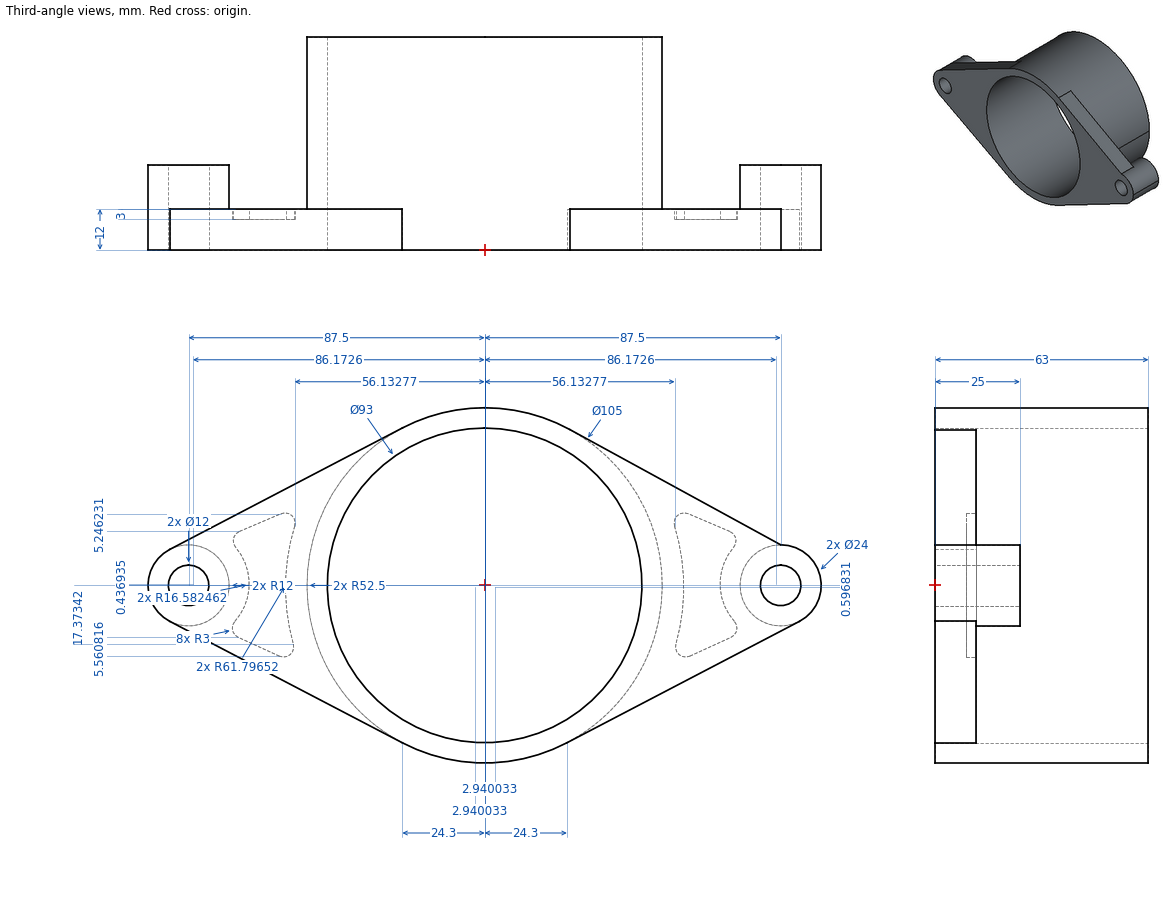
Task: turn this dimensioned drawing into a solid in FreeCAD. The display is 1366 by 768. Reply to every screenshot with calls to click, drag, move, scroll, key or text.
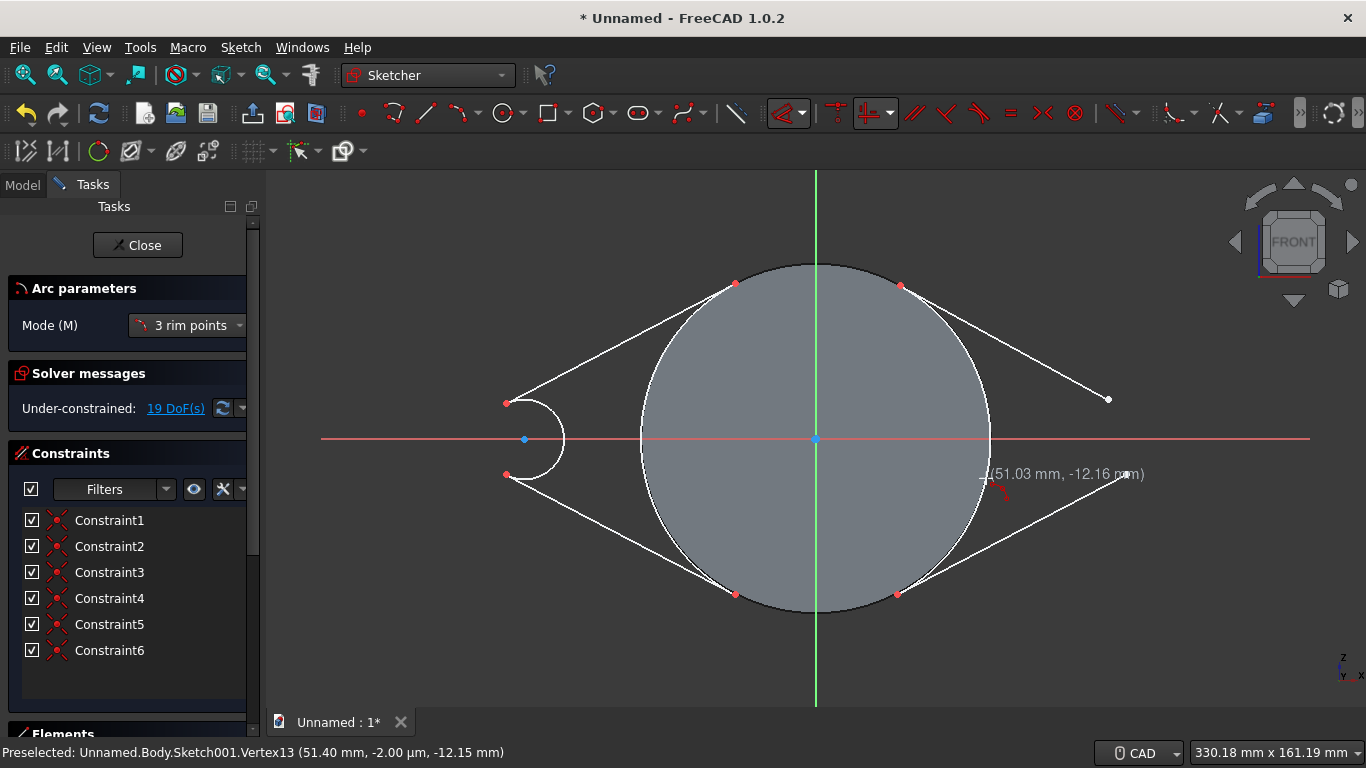
click(1108, 400)
click(1126, 475)
click(1075, 461)
key(Escape)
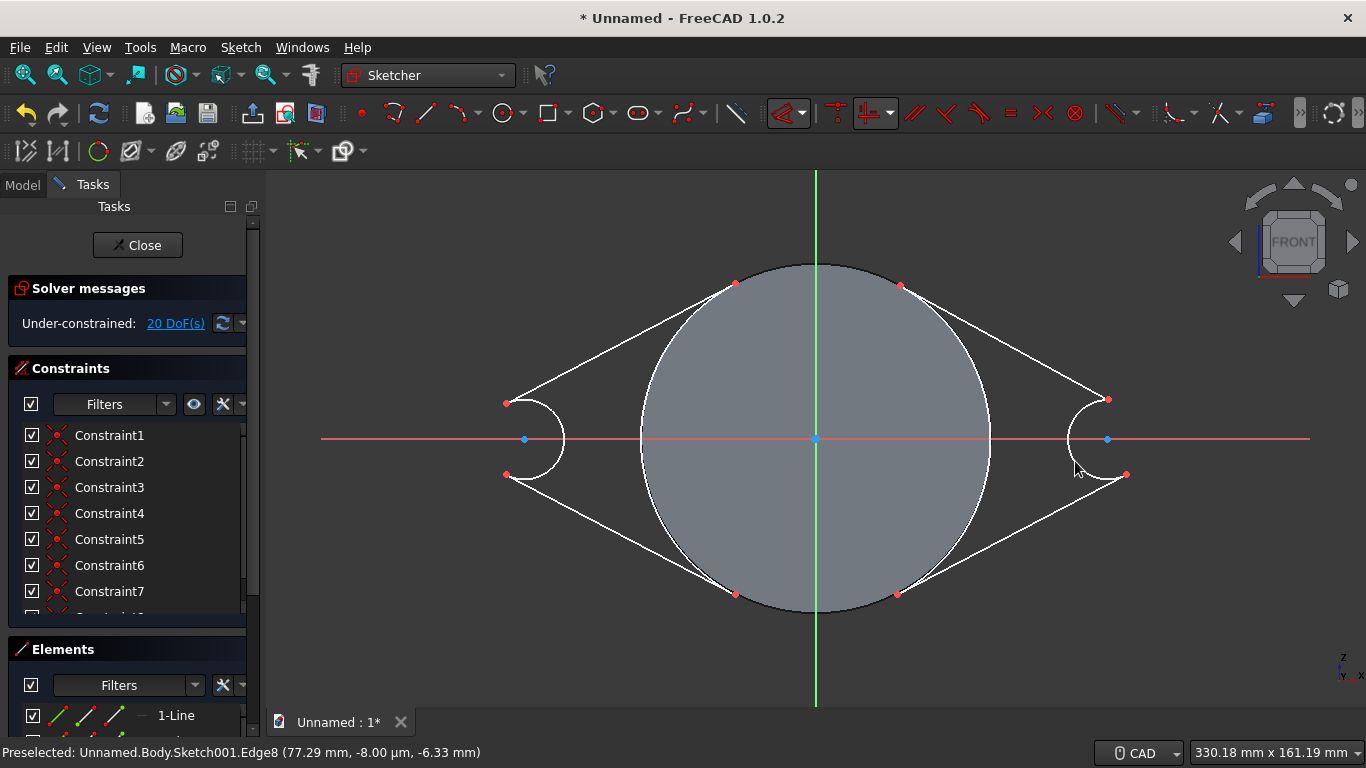
click(666, 559)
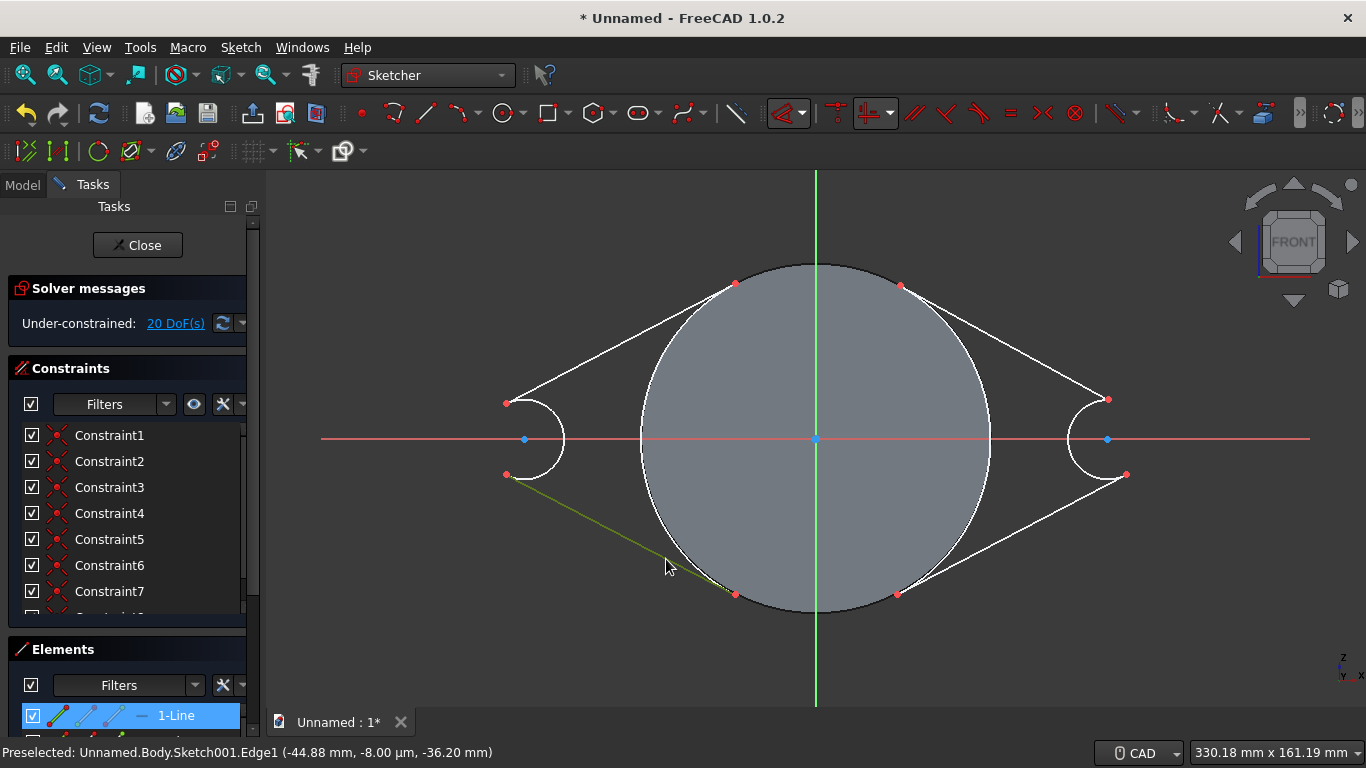
click(552, 469)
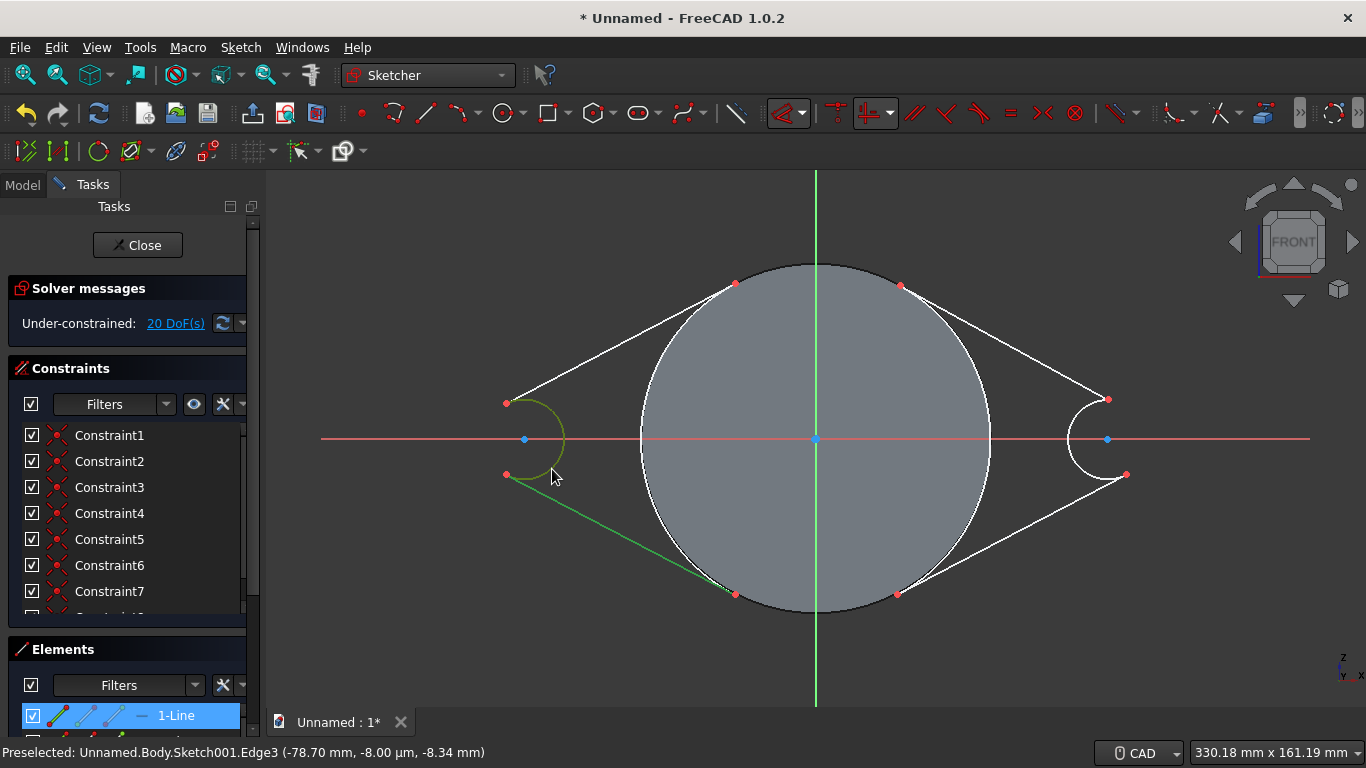
click(980, 114)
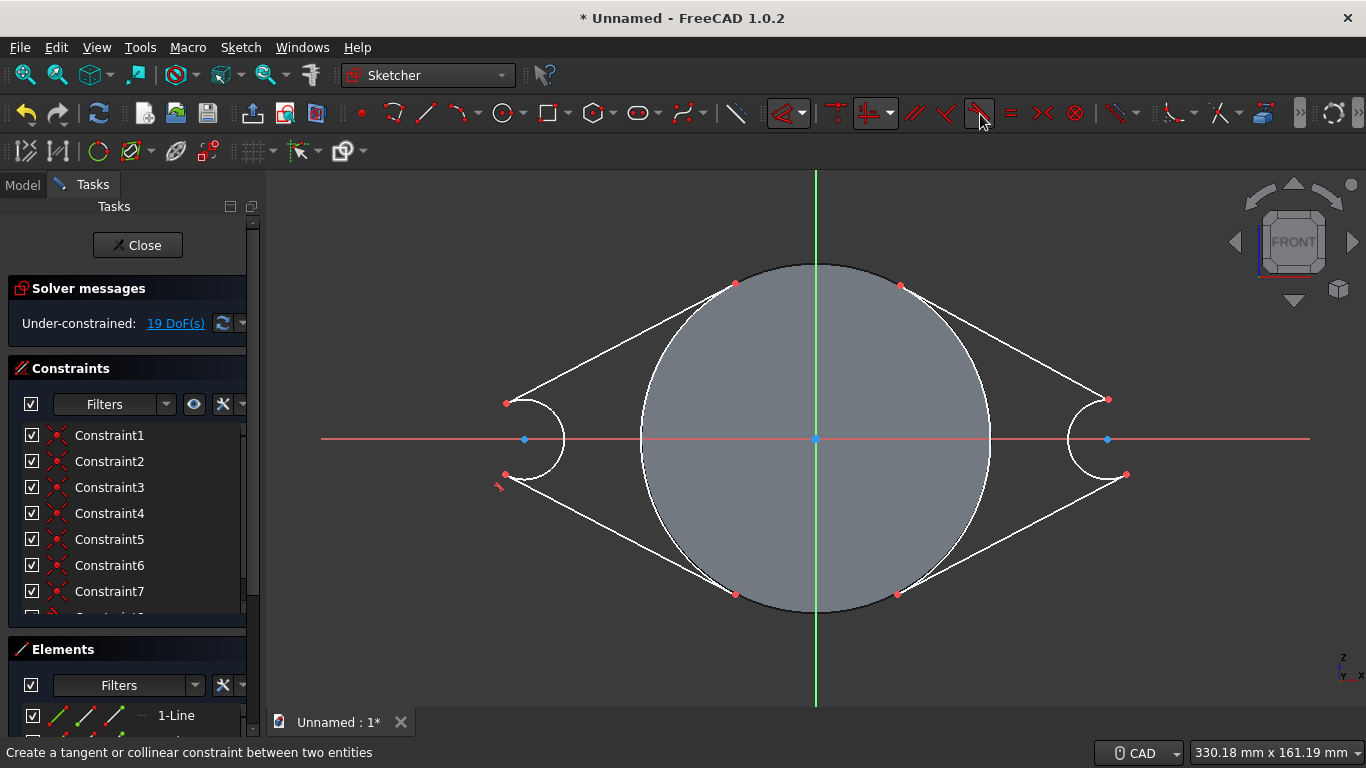
click(666, 559)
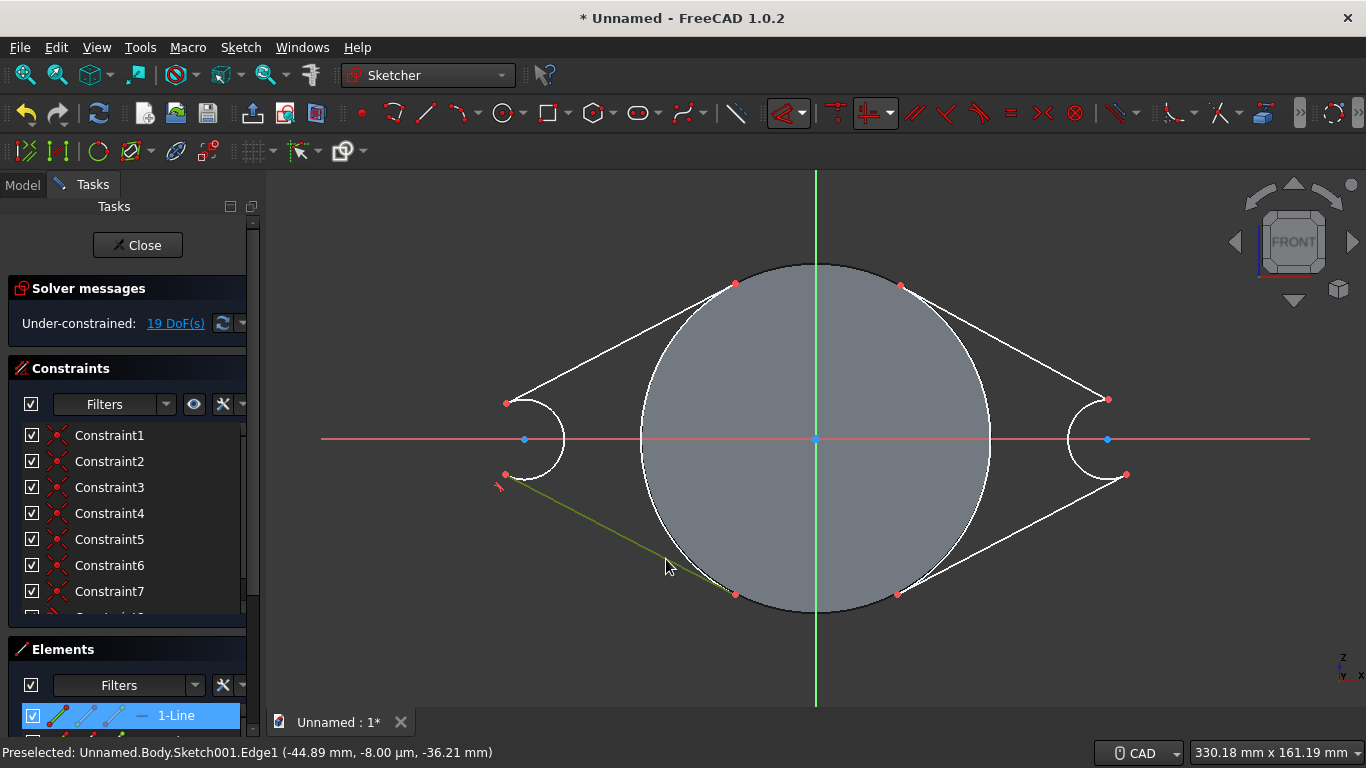
click(657, 365)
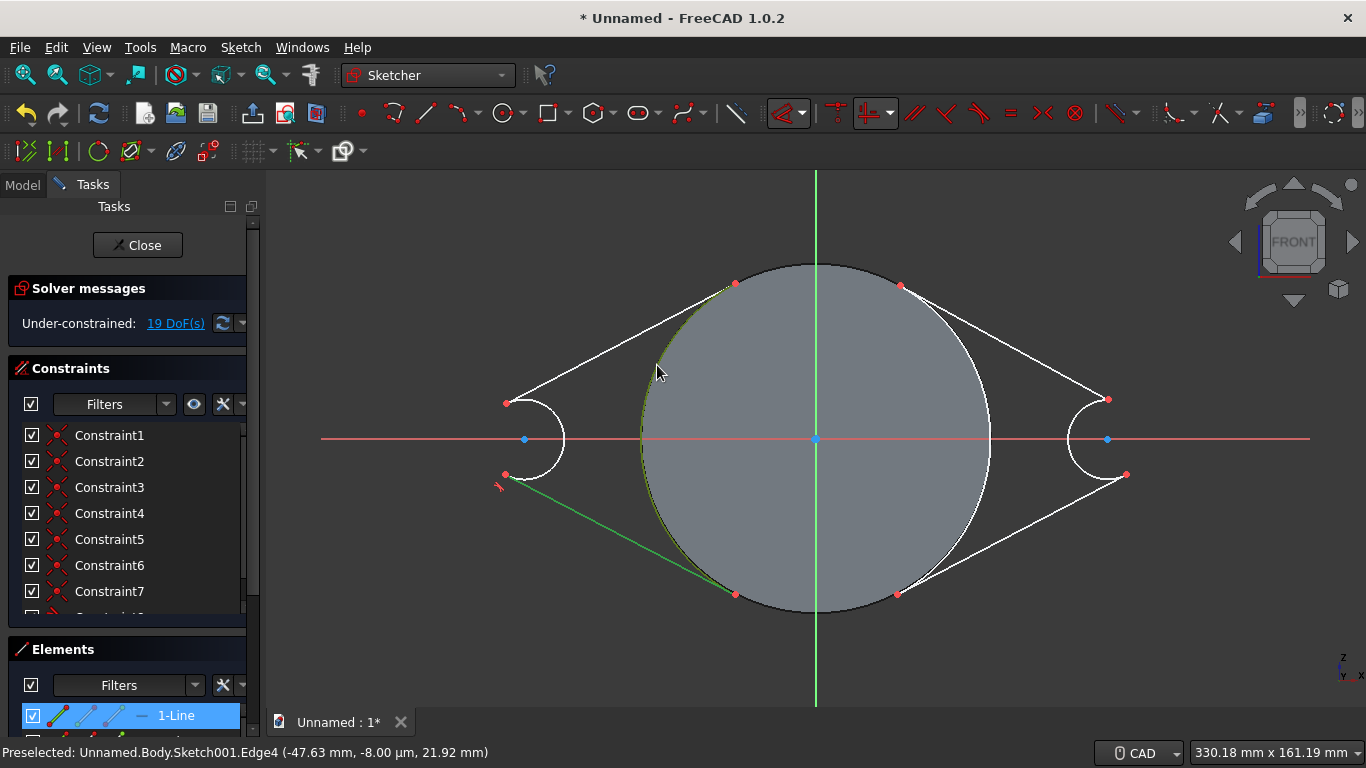
key(t)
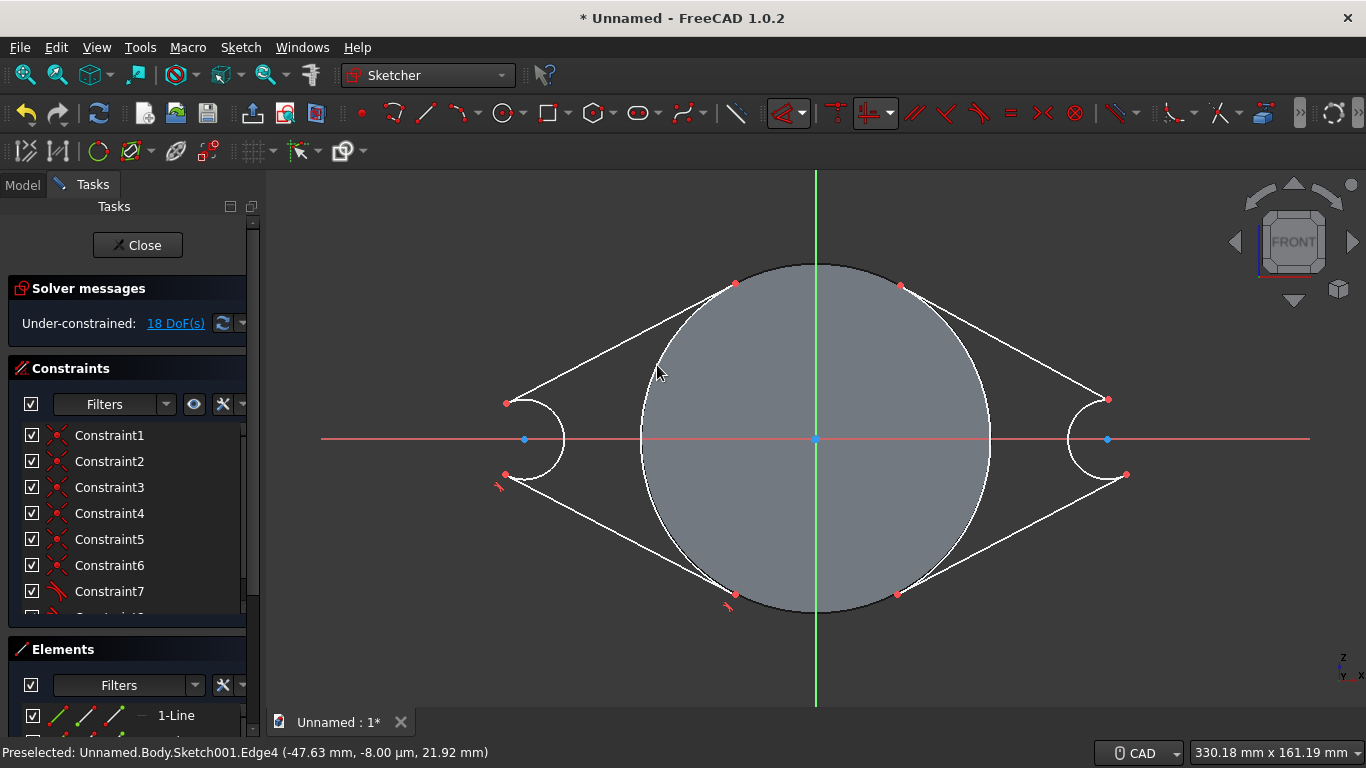
click(575, 368)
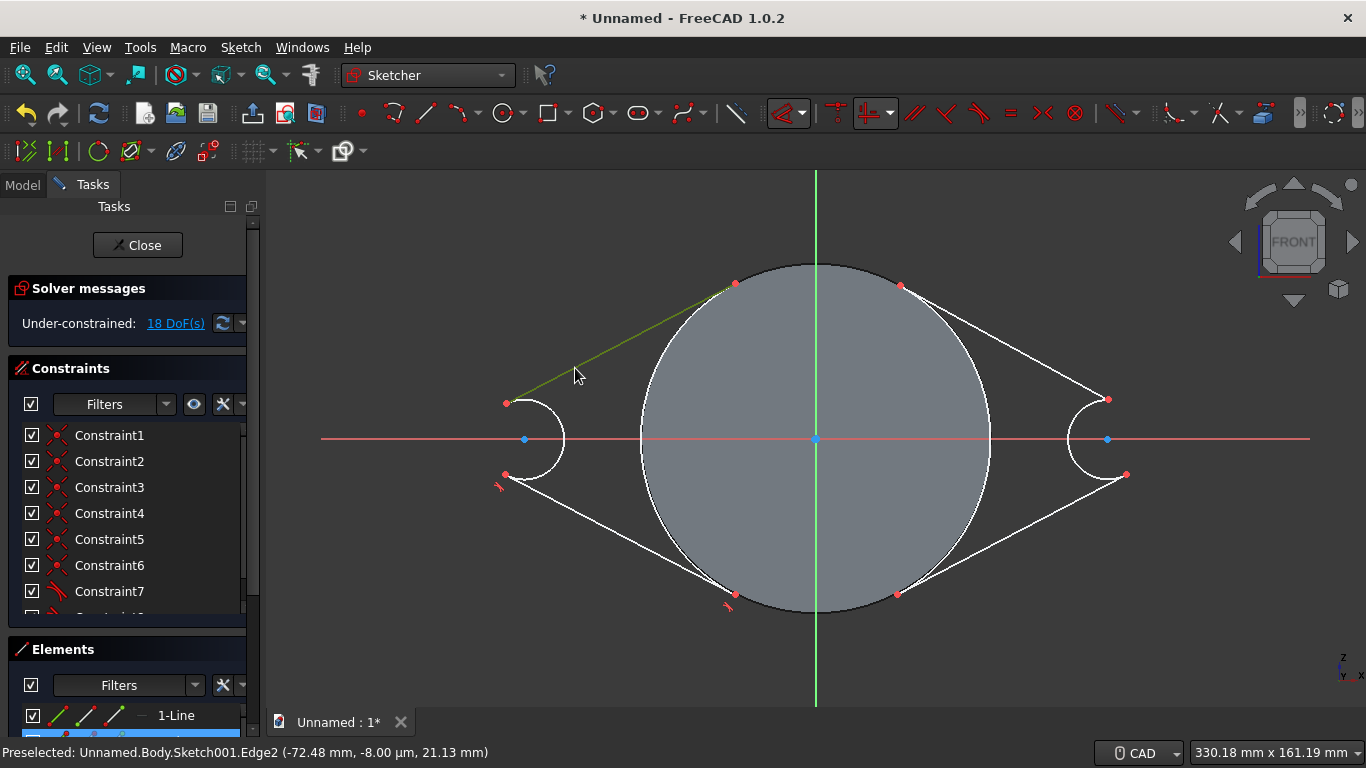
click(551, 469)